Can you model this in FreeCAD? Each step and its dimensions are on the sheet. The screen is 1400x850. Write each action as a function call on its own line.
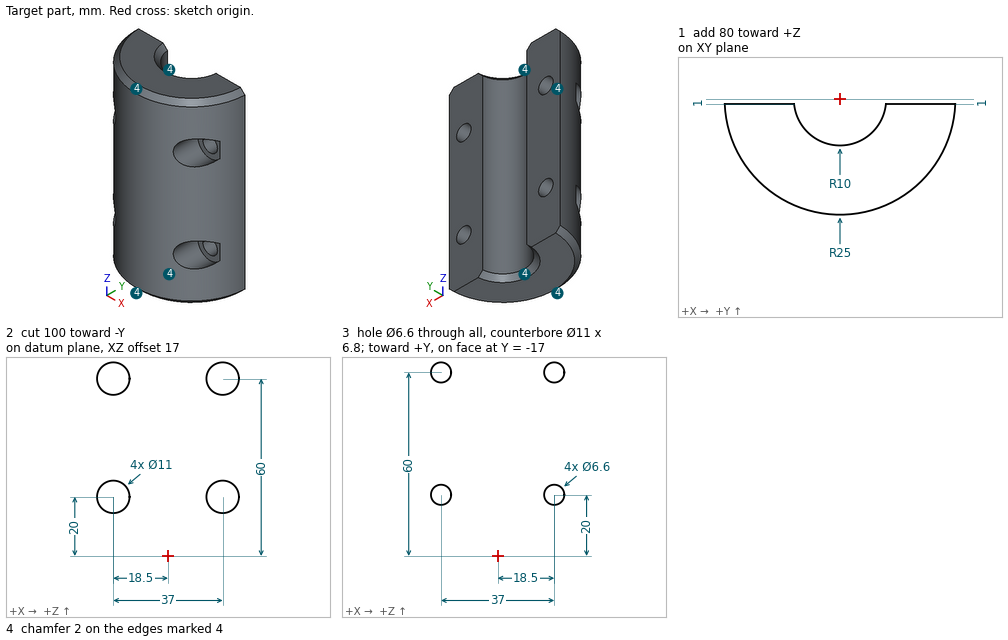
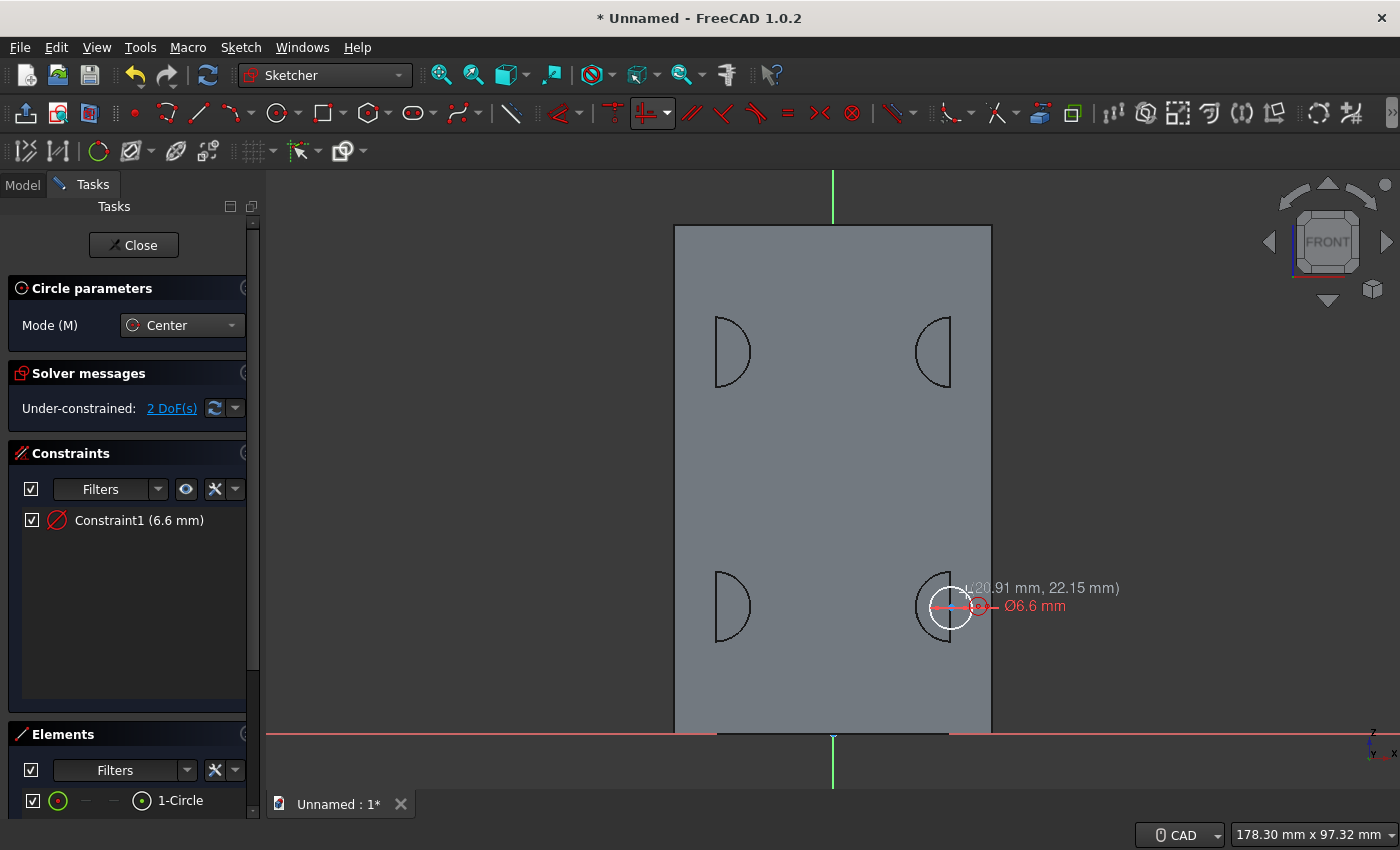
click(715, 607)
move(730, 592)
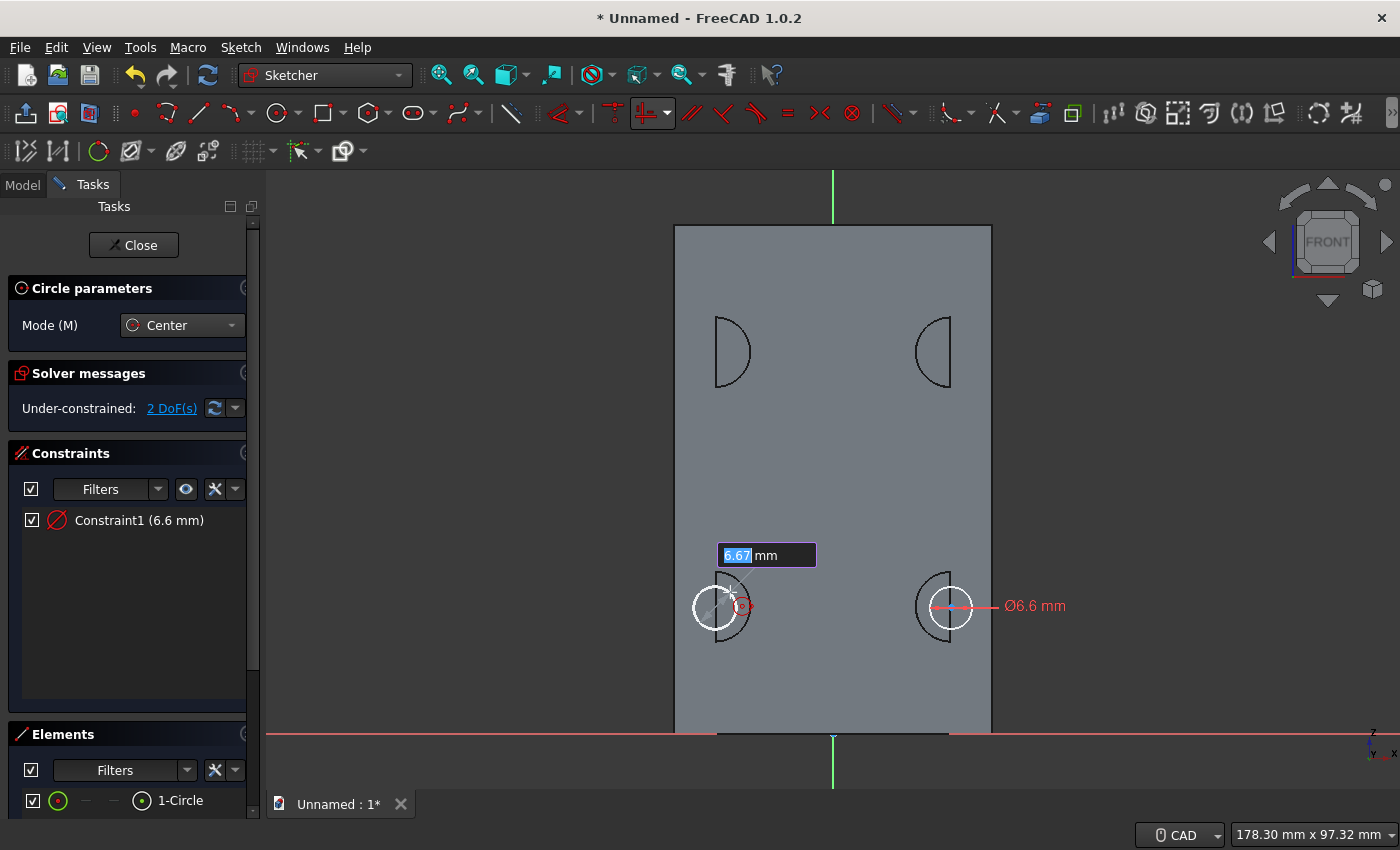
text(6.6)
key(Return)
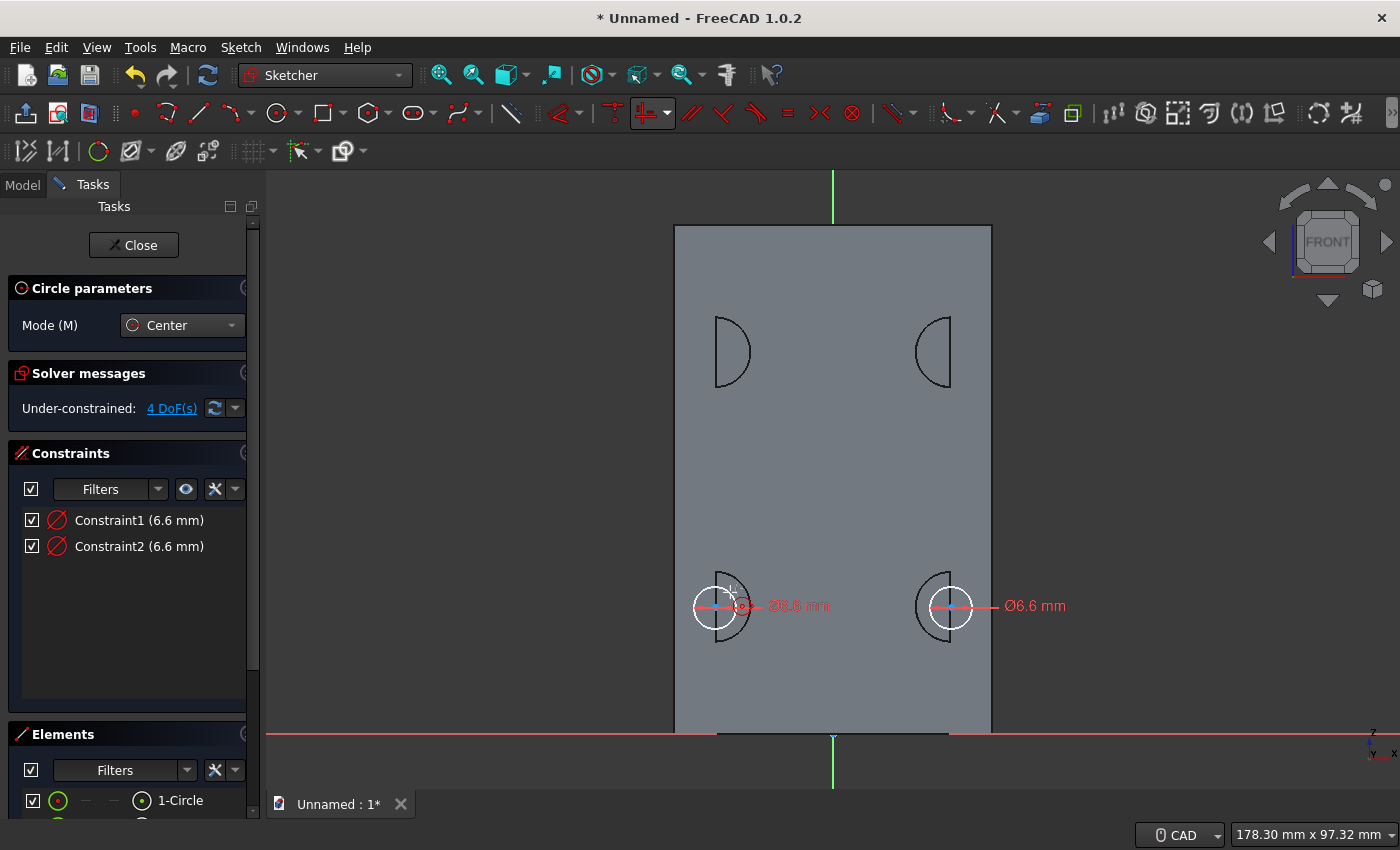
click(715, 352)
move(730, 337)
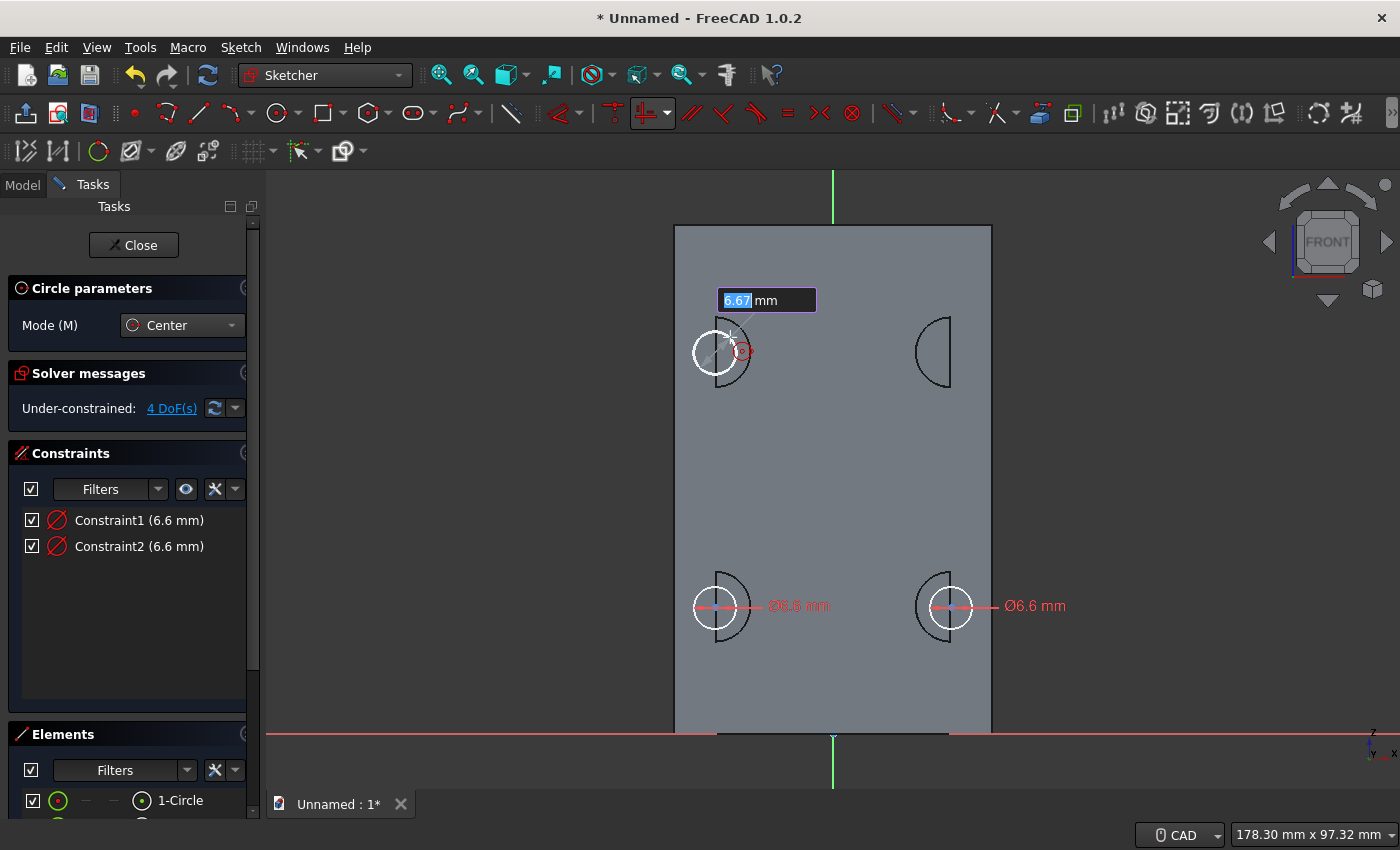
text(6.6)
key(Return)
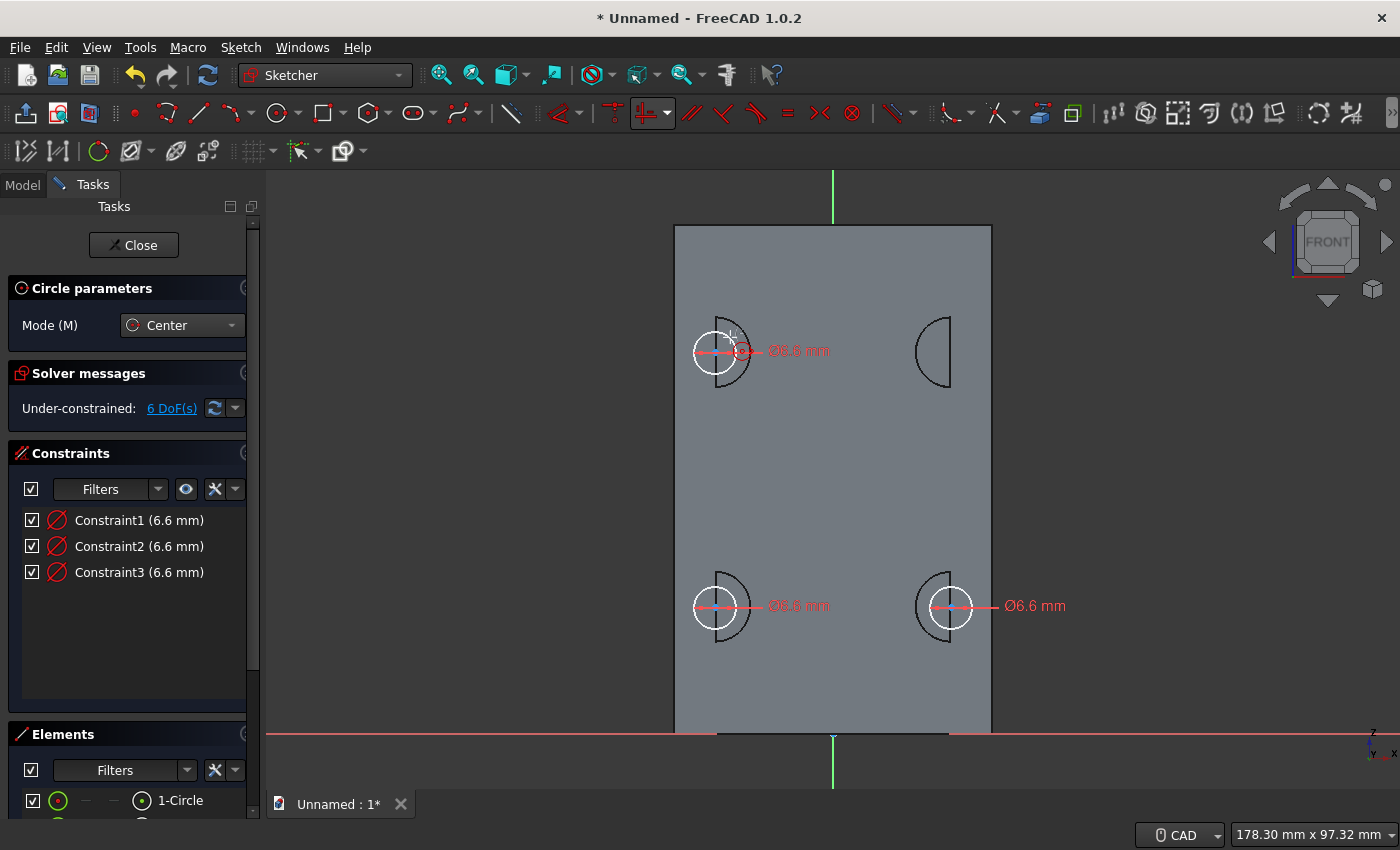
click(951, 352)
move(966, 337)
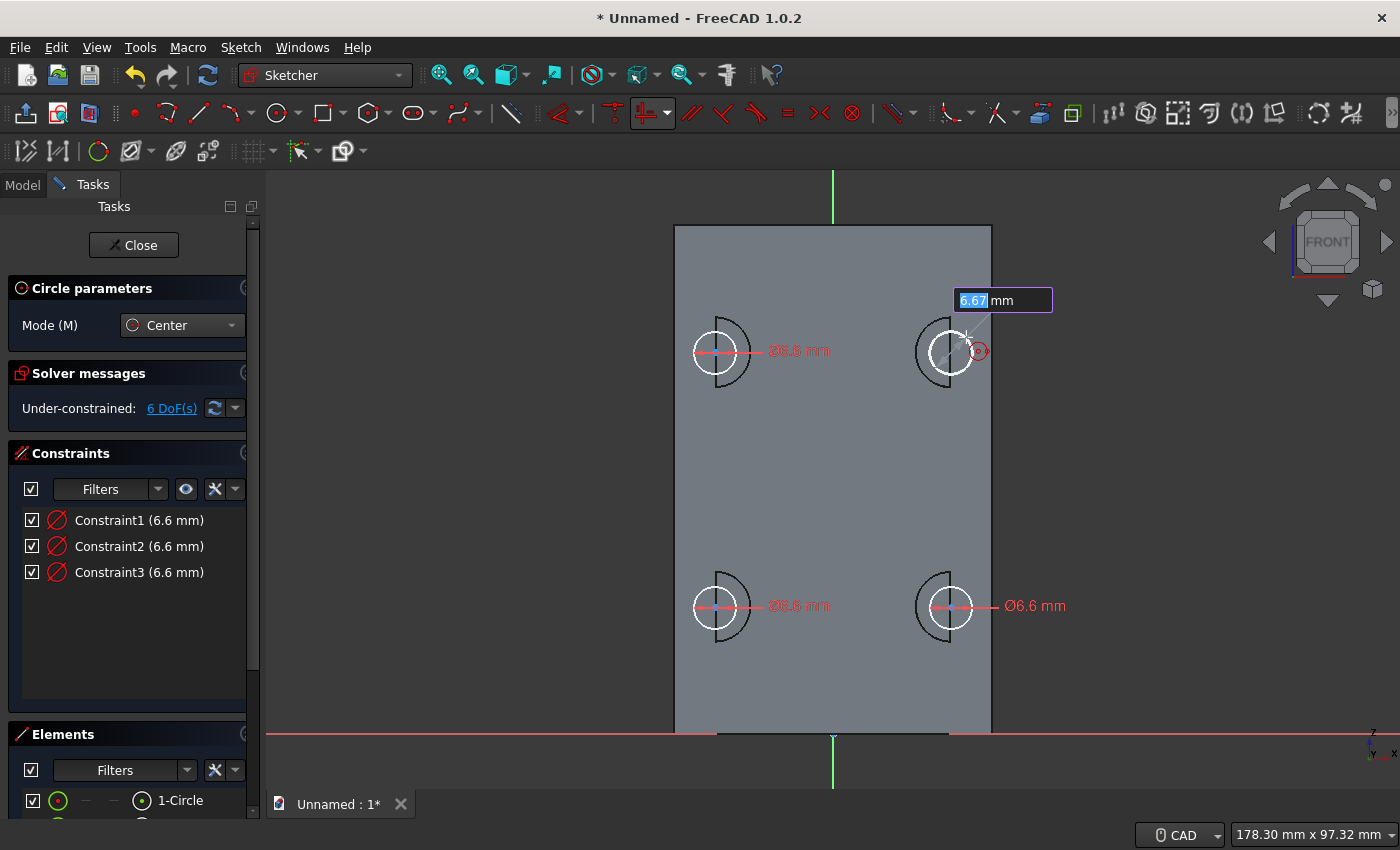
text(6.6)
key(Return)
key(Escape)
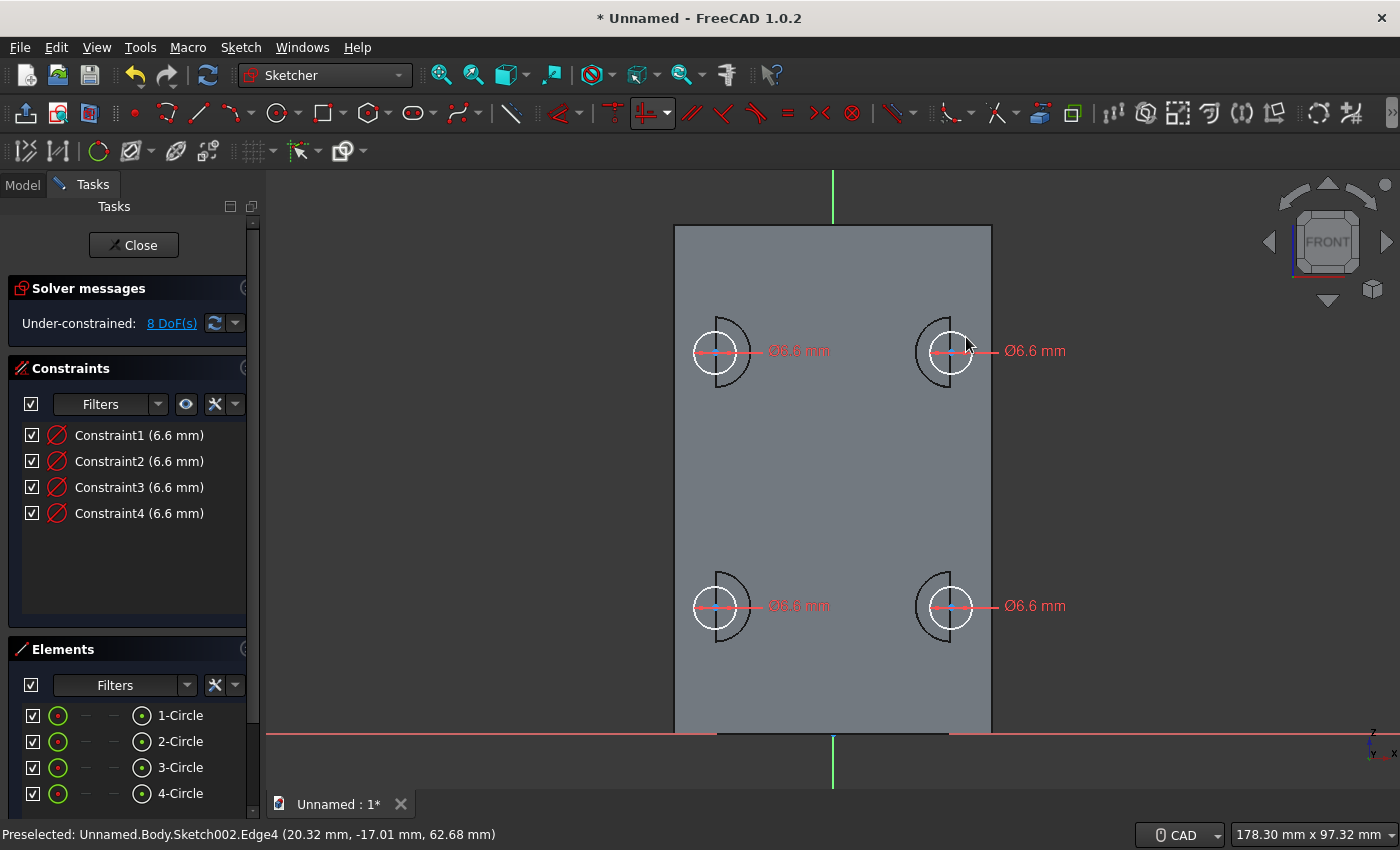
click(951, 608)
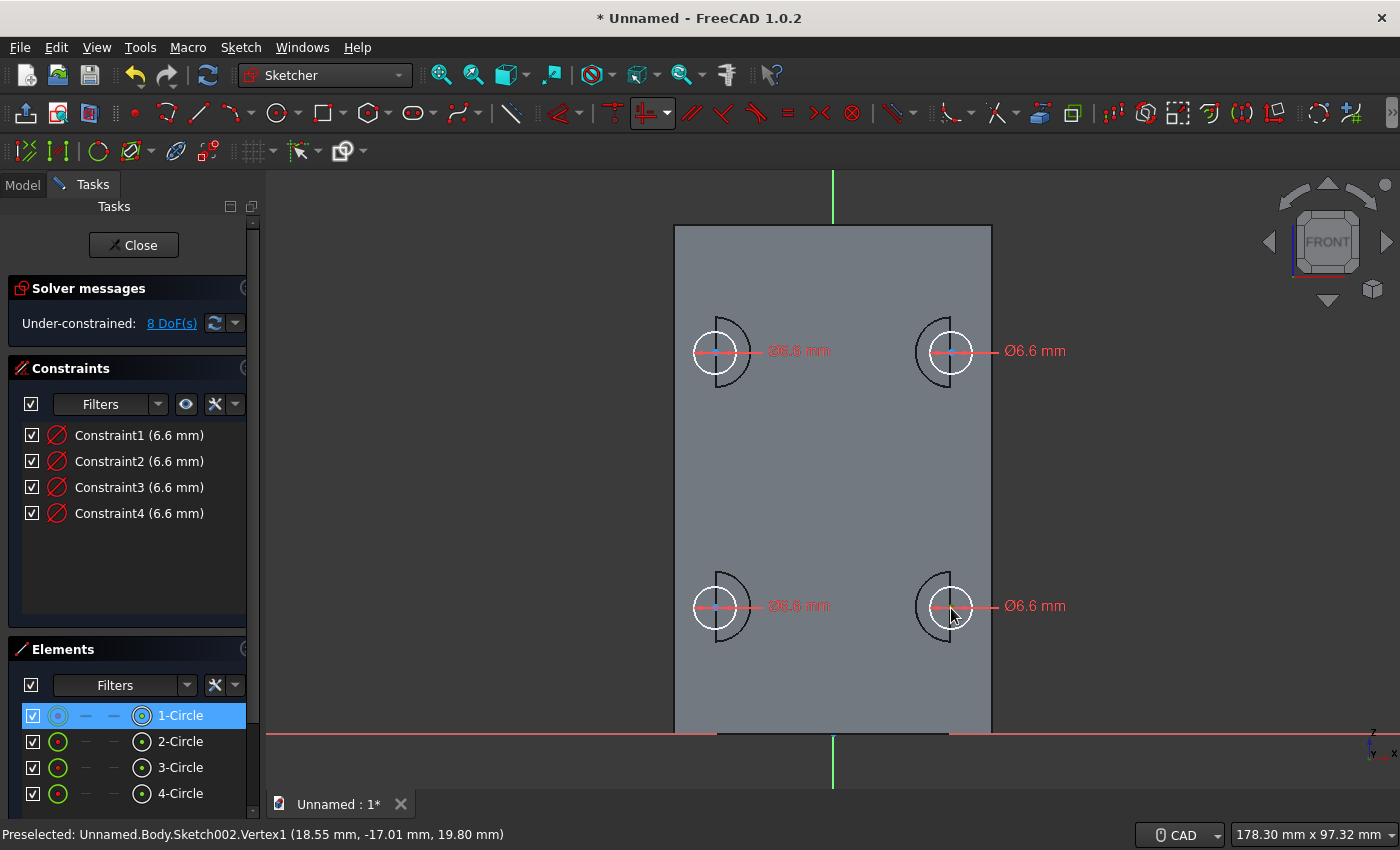
click(715, 608)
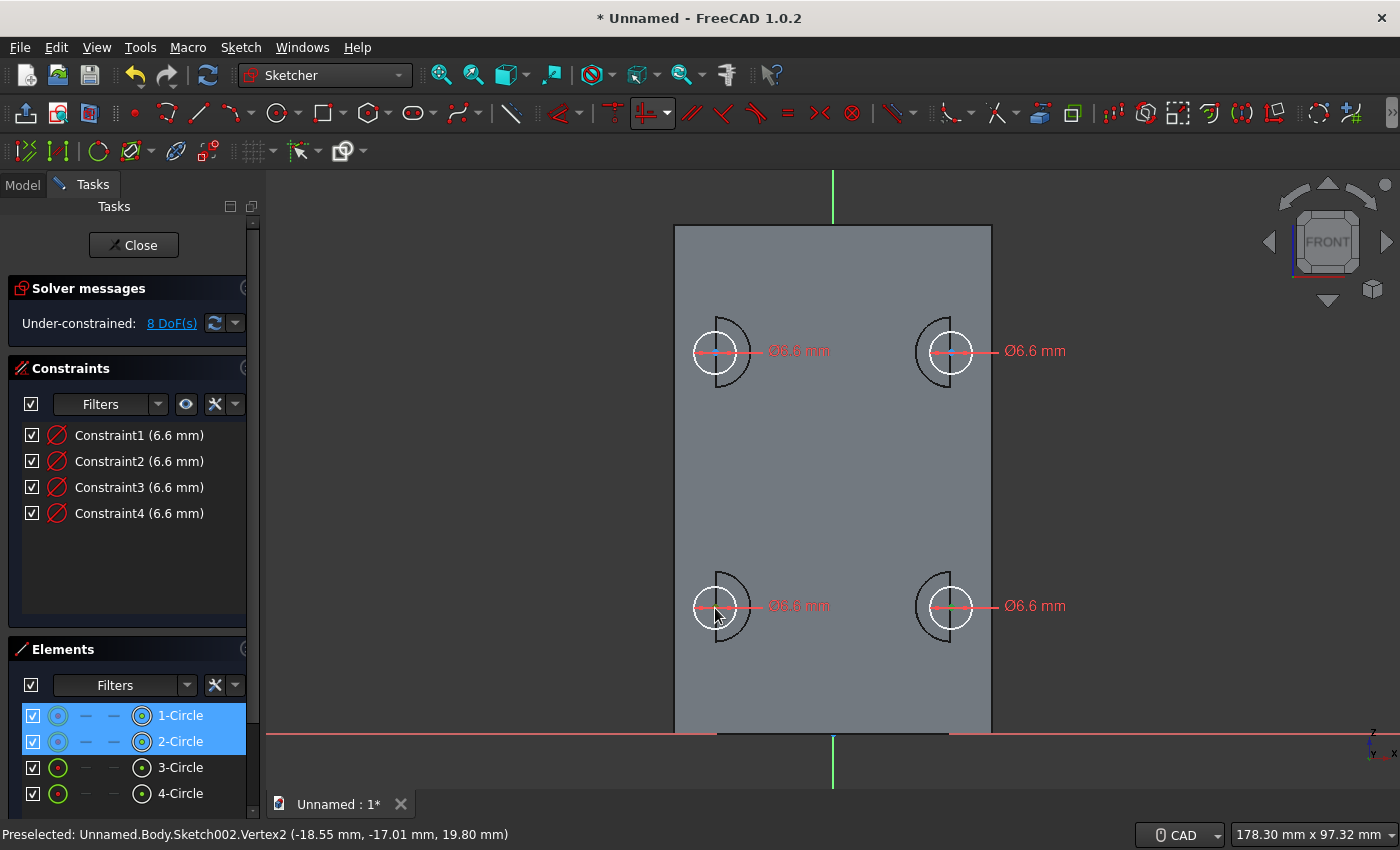
key(h)